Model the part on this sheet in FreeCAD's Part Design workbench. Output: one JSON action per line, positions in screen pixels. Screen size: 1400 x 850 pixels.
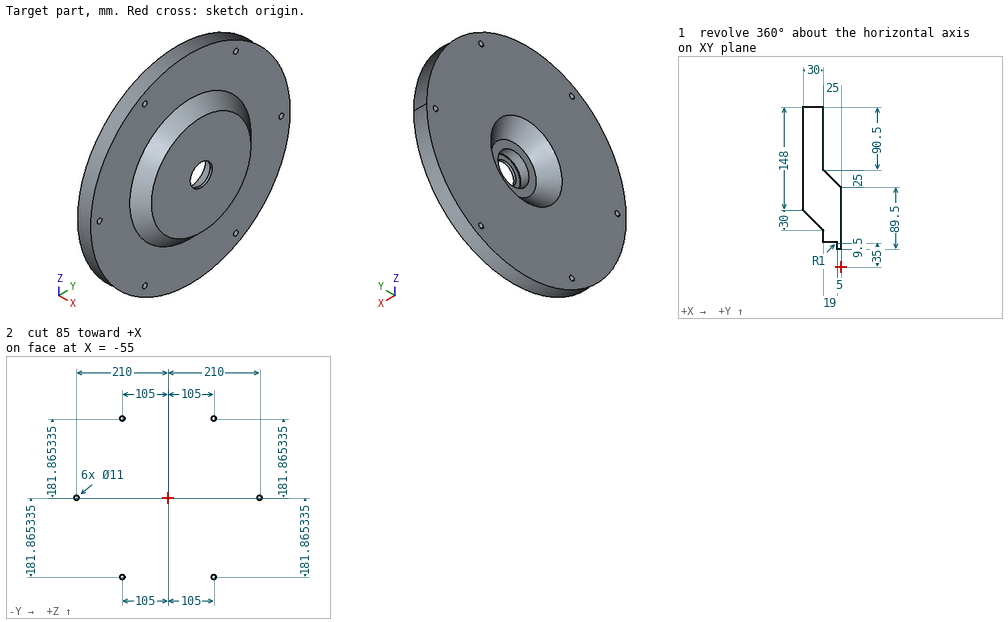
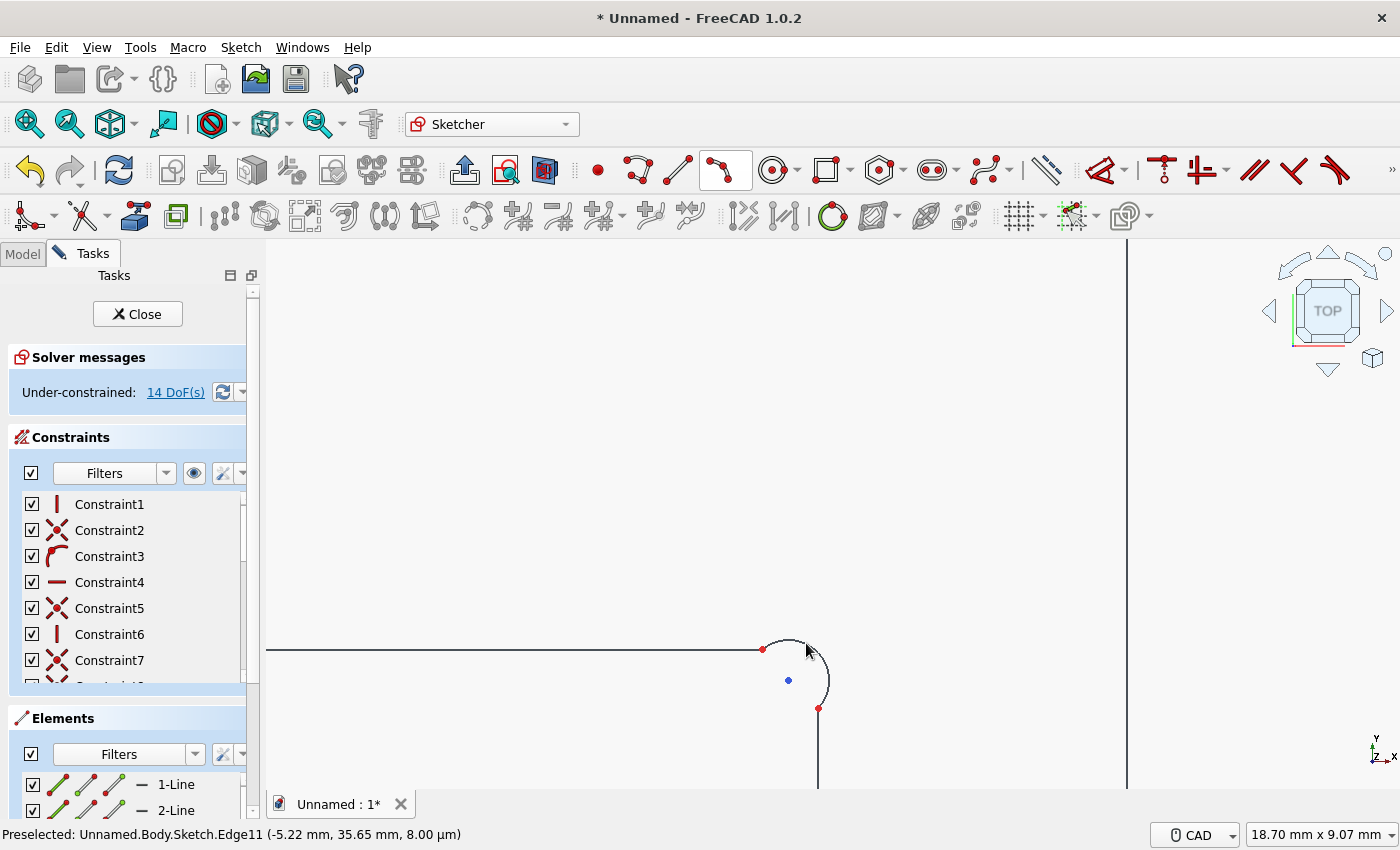
{"action": "scroll", "coordinate": [801, 646], "scroll_direction": "down", "scroll_amount": 18}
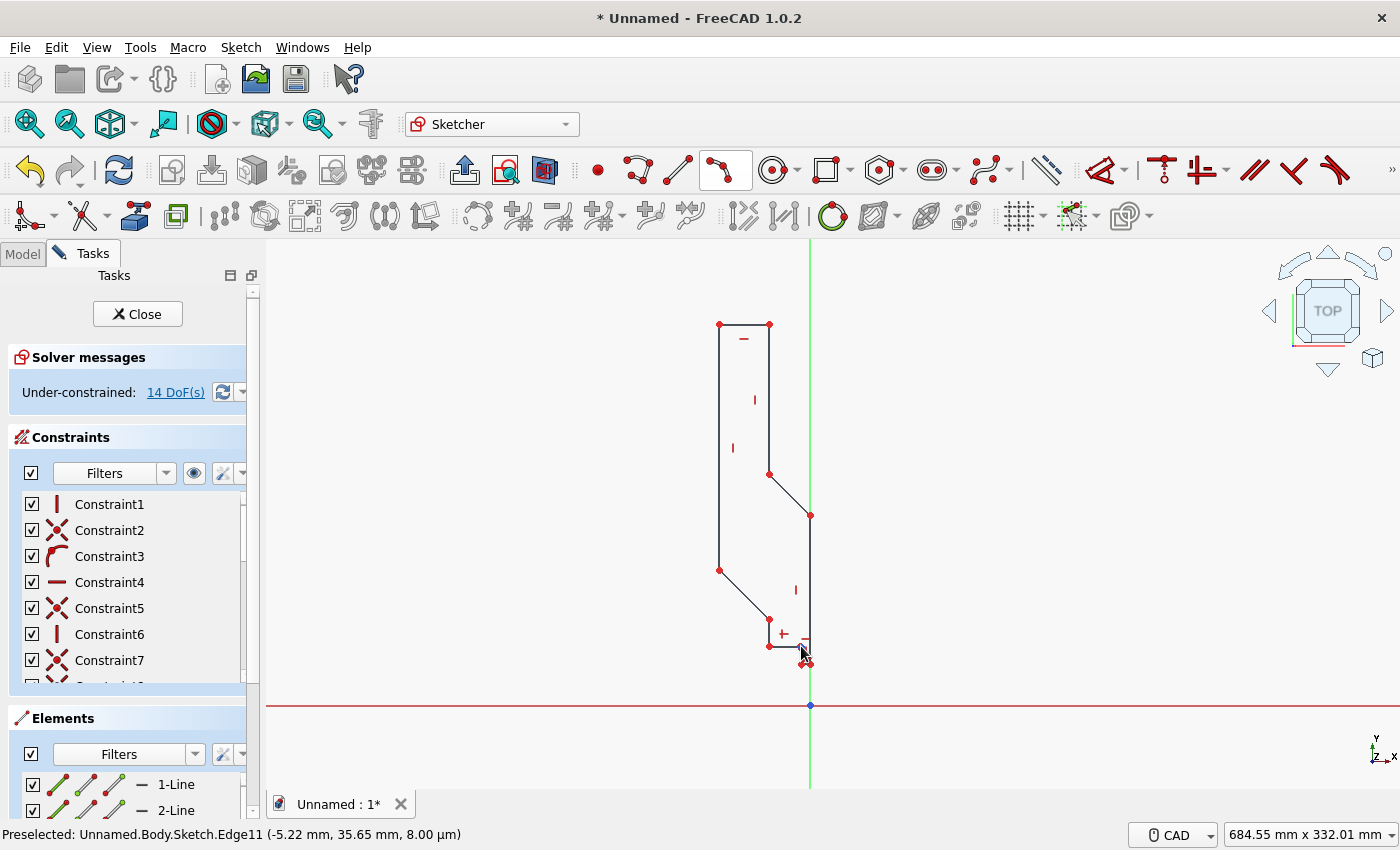
{"action": "scroll", "coordinate": [802, 653], "scroll_direction": "up", "scroll_amount": 6}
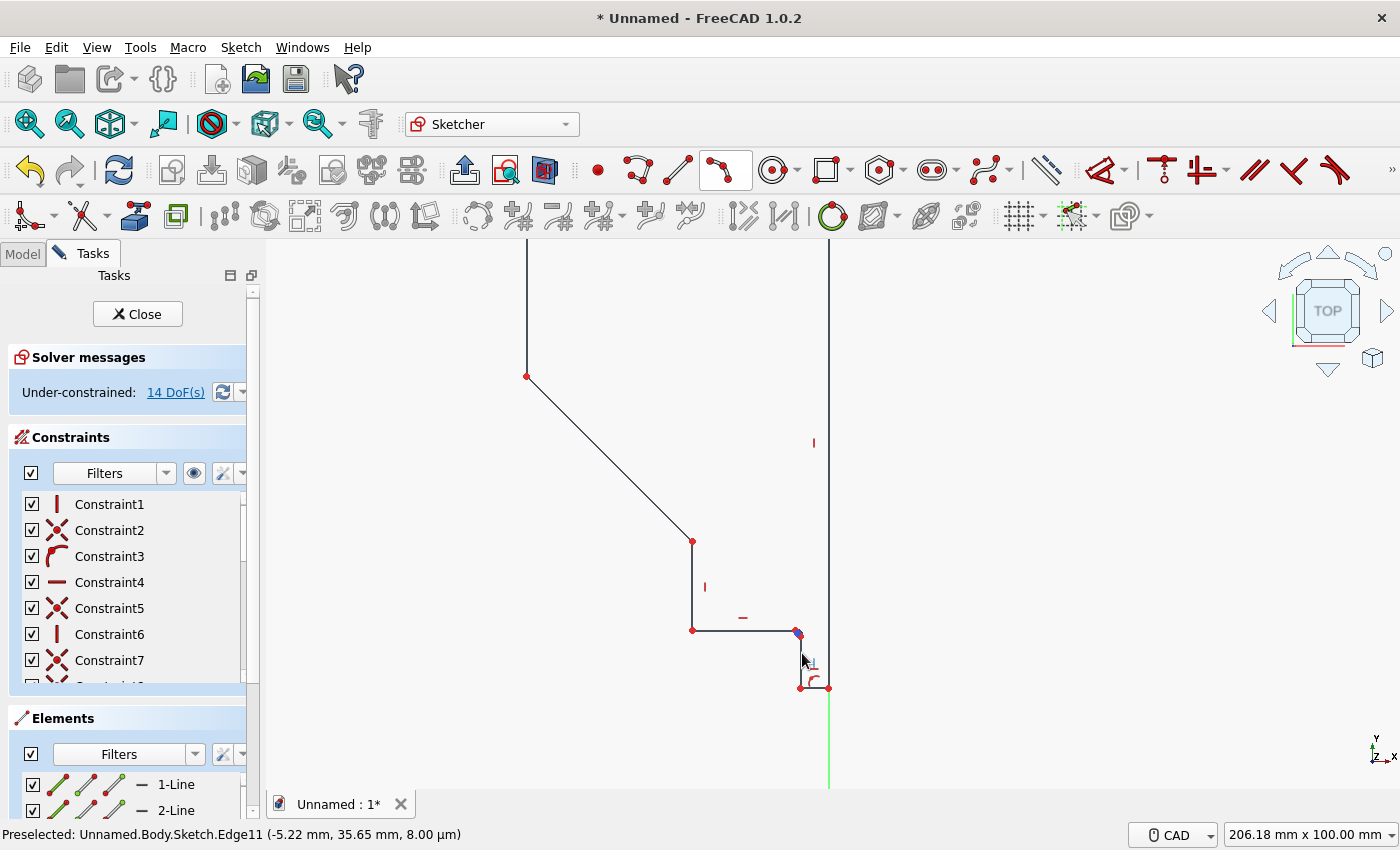
{"action": "left_click", "coordinate": [801, 652]}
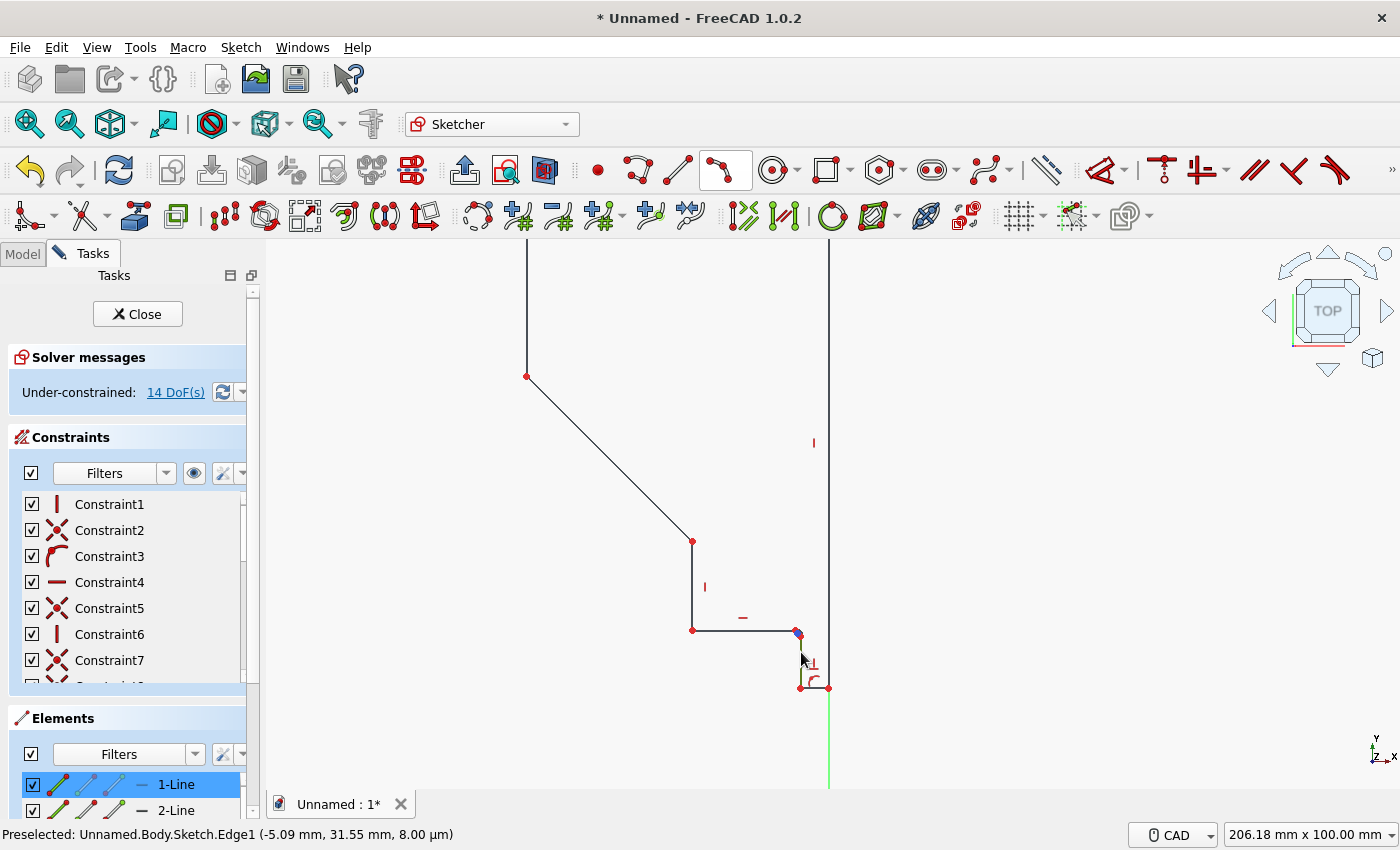
{"action": "scroll", "coordinate": [801, 631], "scroll_direction": "up", "scroll_amount": 7}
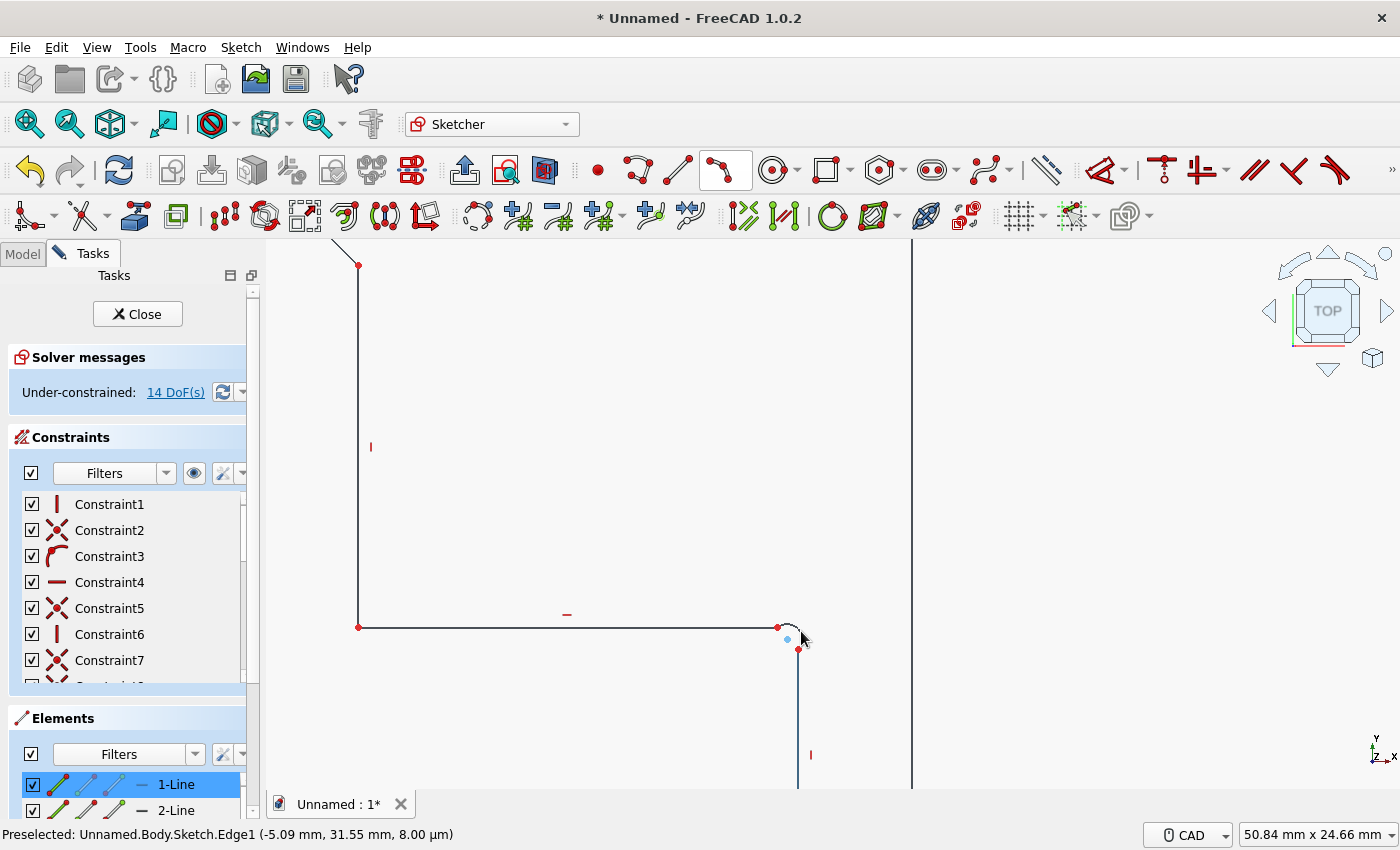
{"action": "left_click", "coordinate": [798, 629]}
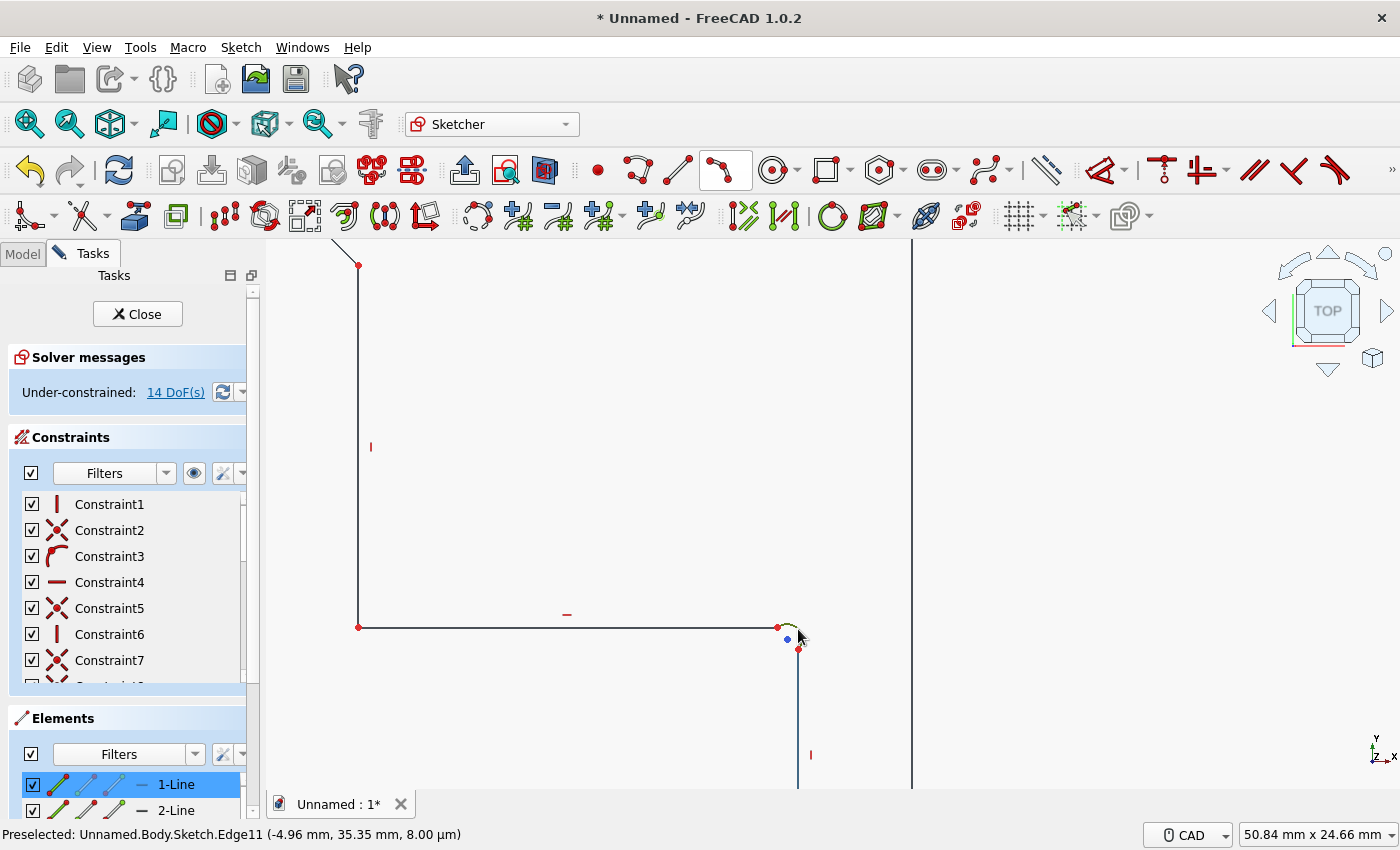
{"action": "left_click", "coordinate": [1336, 170]}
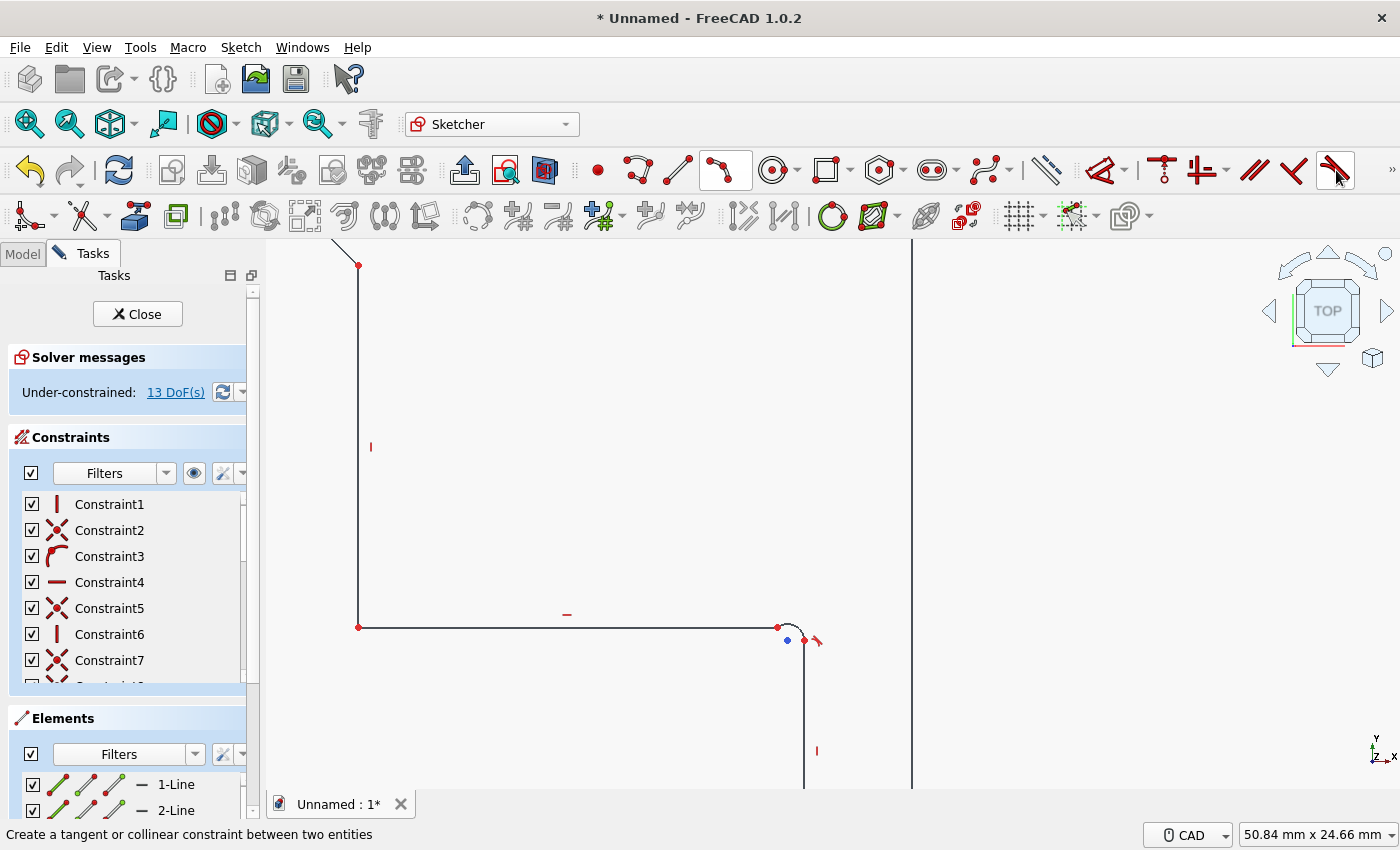
{"action": "scroll", "coordinate": [802, 647], "scroll_direction": "down", "scroll_amount": 13}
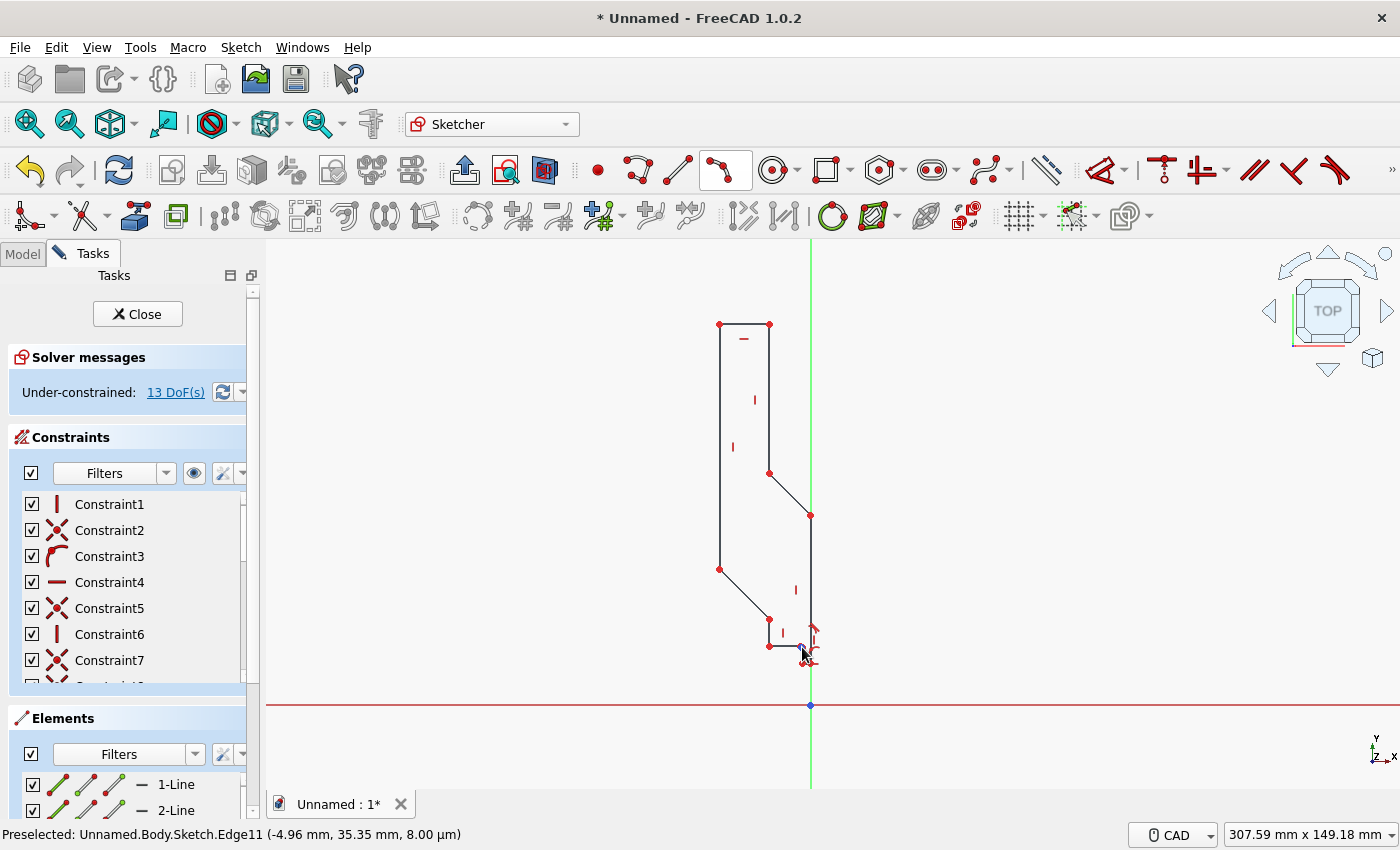
{"action": "scroll", "coordinate": [779, 646], "scroll_direction": "up", "scroll_amount": 2}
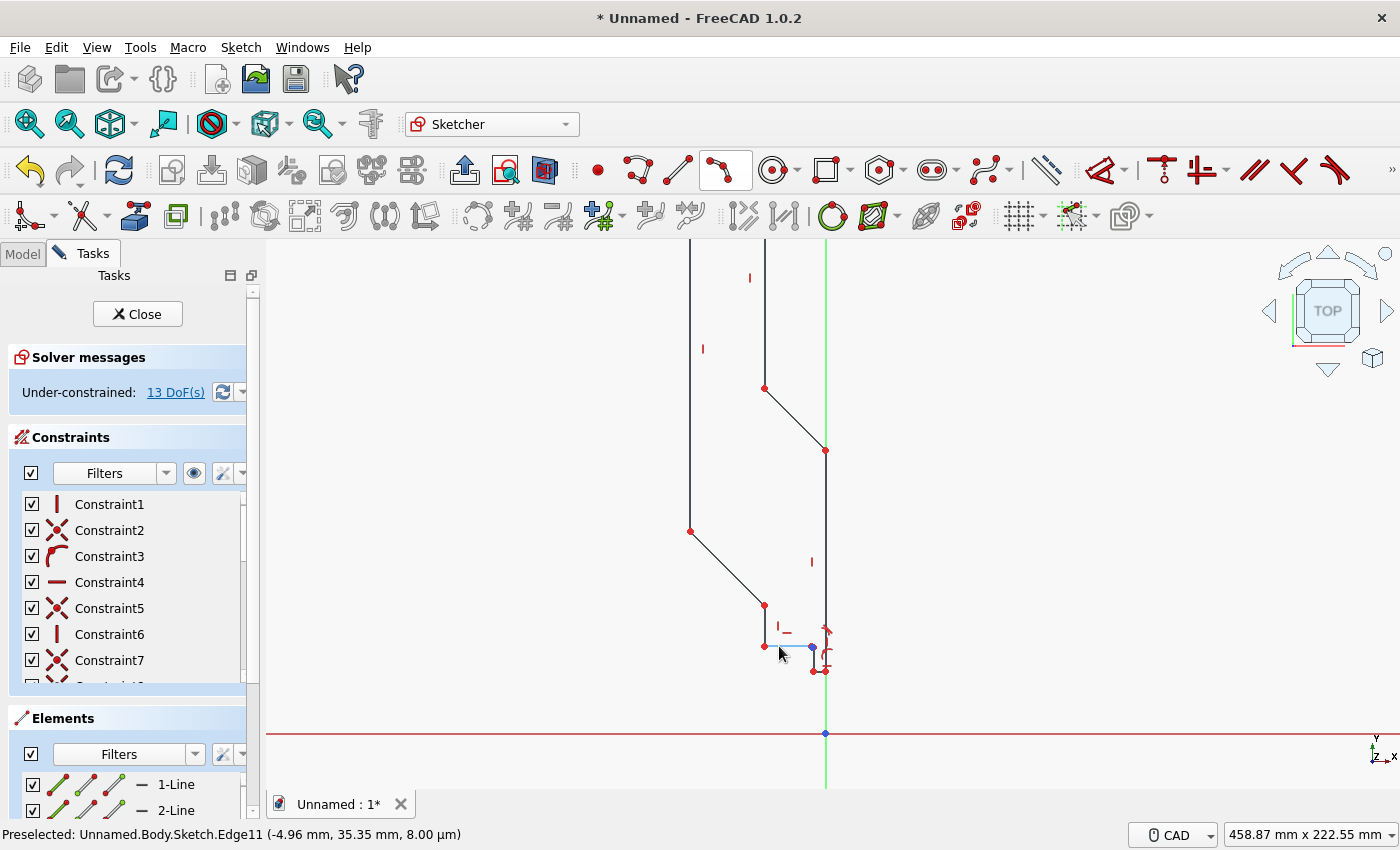
{"action": "left_click", "coordinate": [778, 646]}